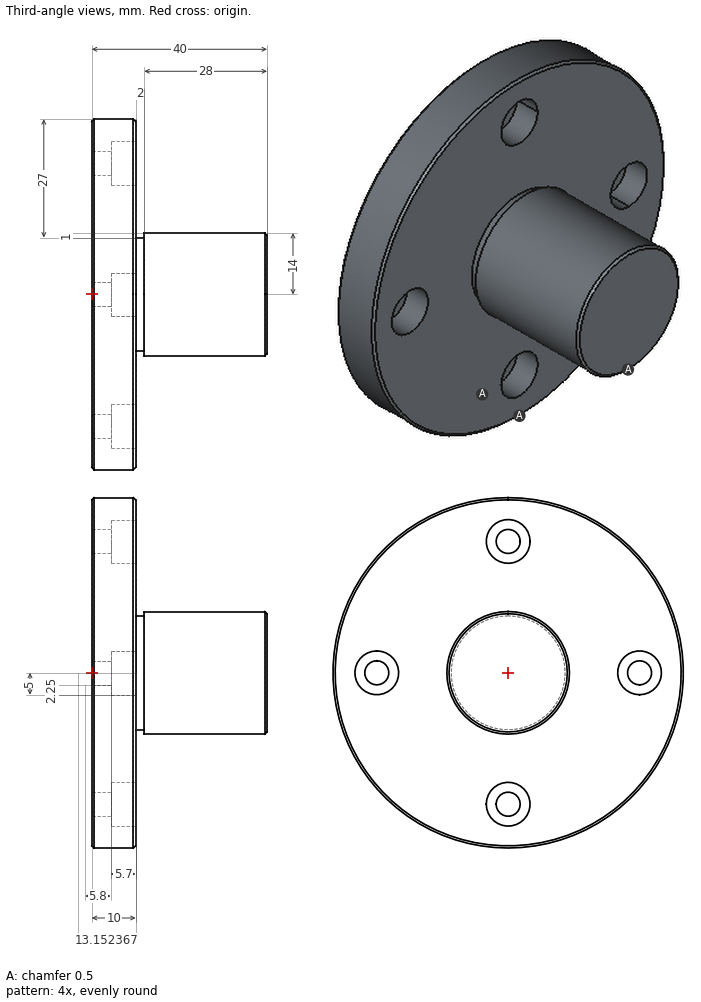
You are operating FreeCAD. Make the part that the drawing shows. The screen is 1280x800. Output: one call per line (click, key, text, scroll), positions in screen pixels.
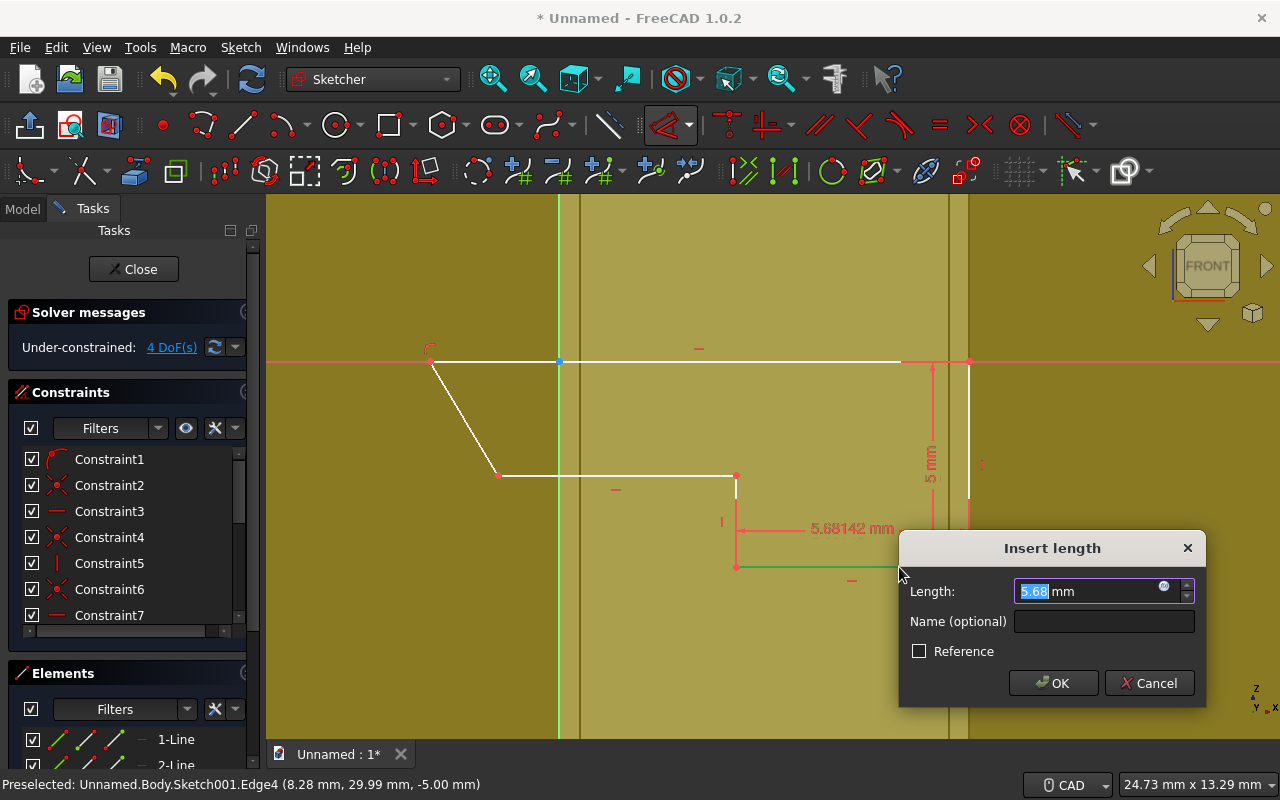
text(5.7)
key(Return)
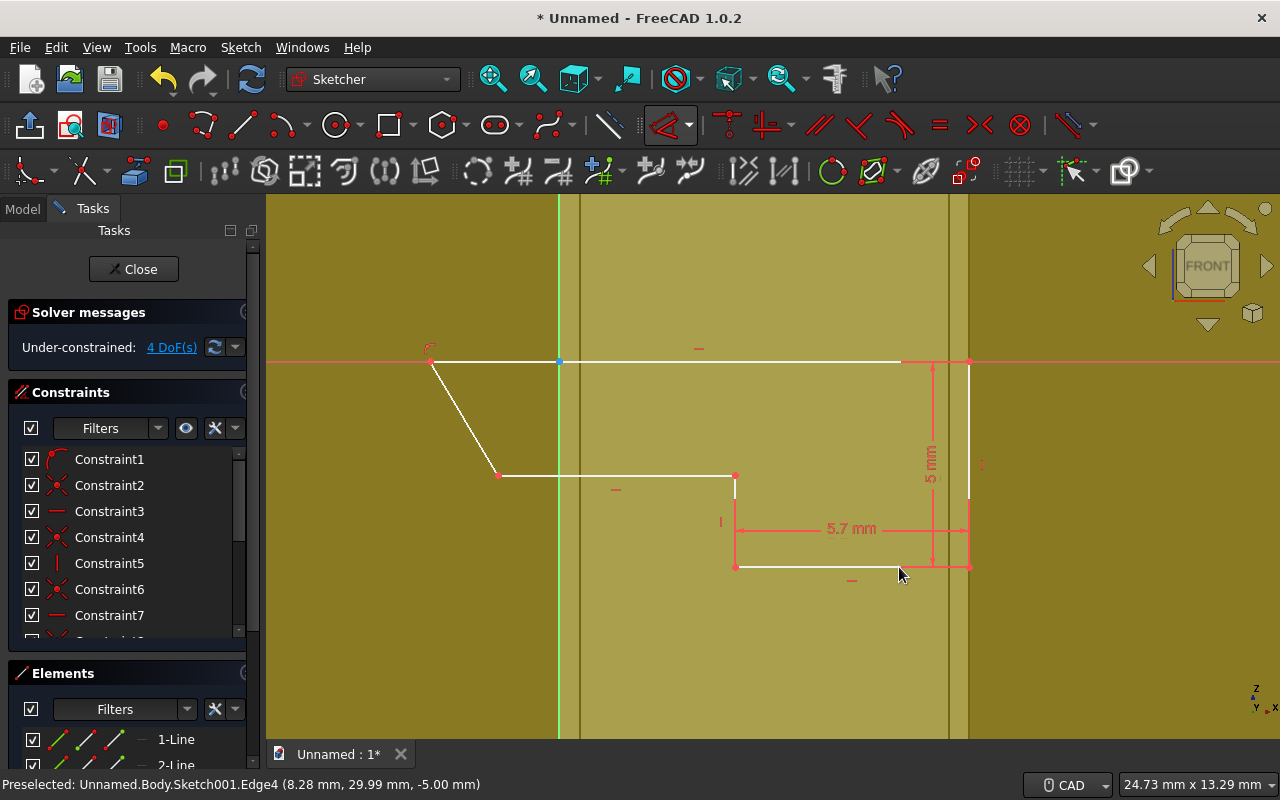
click(664, 476)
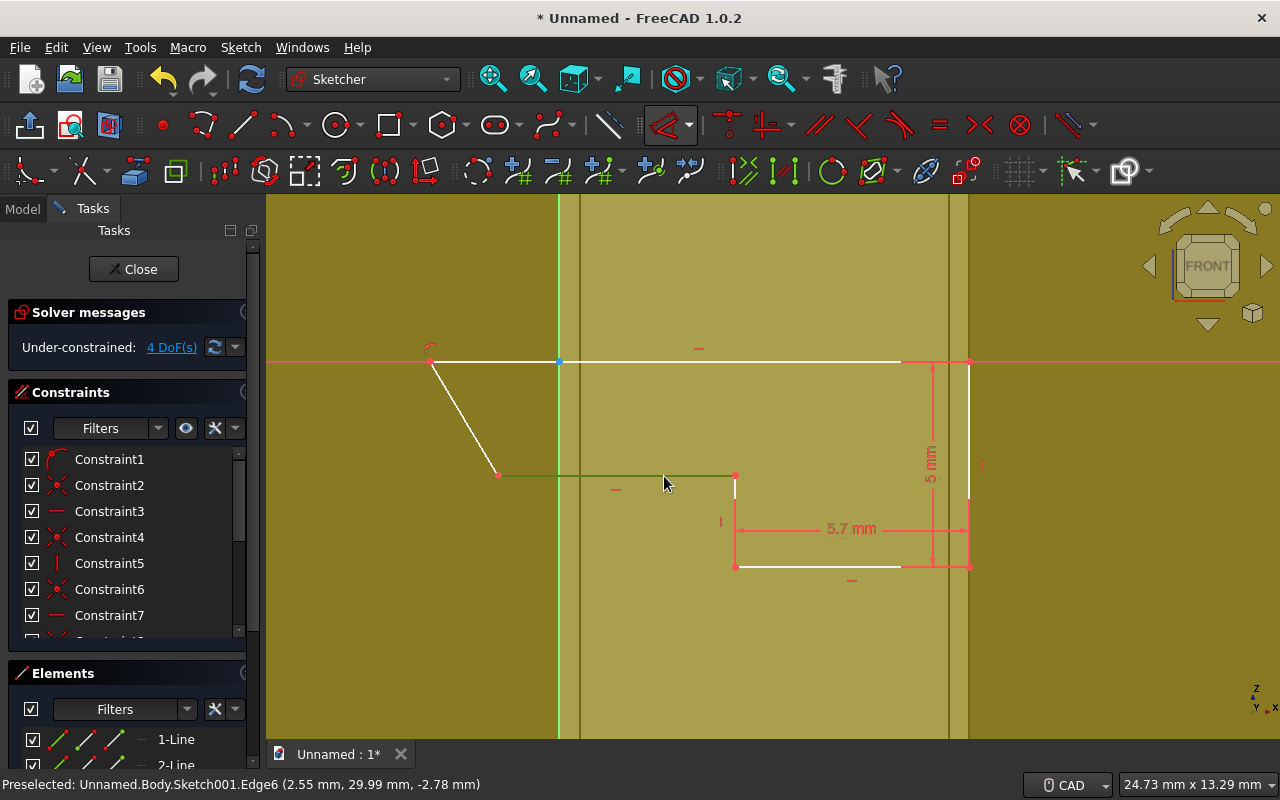
click(692, 126)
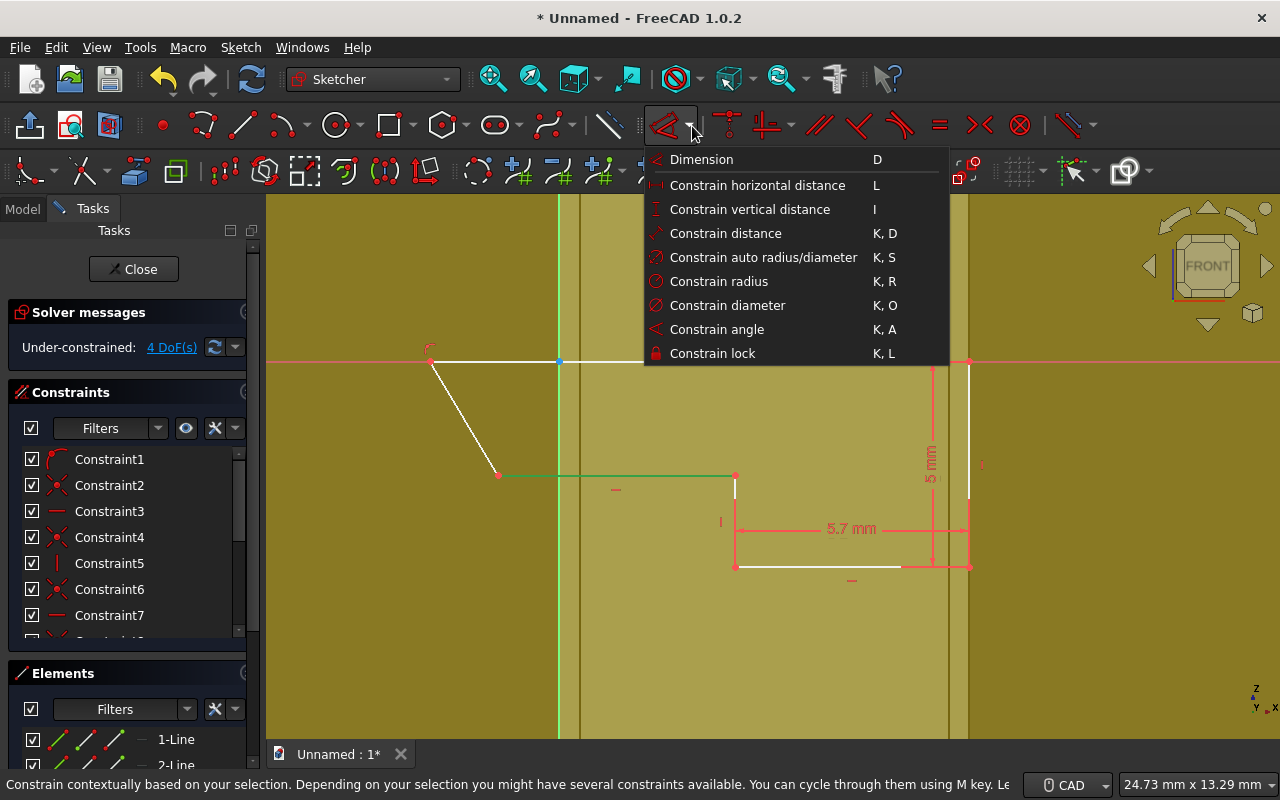
click(797, 185)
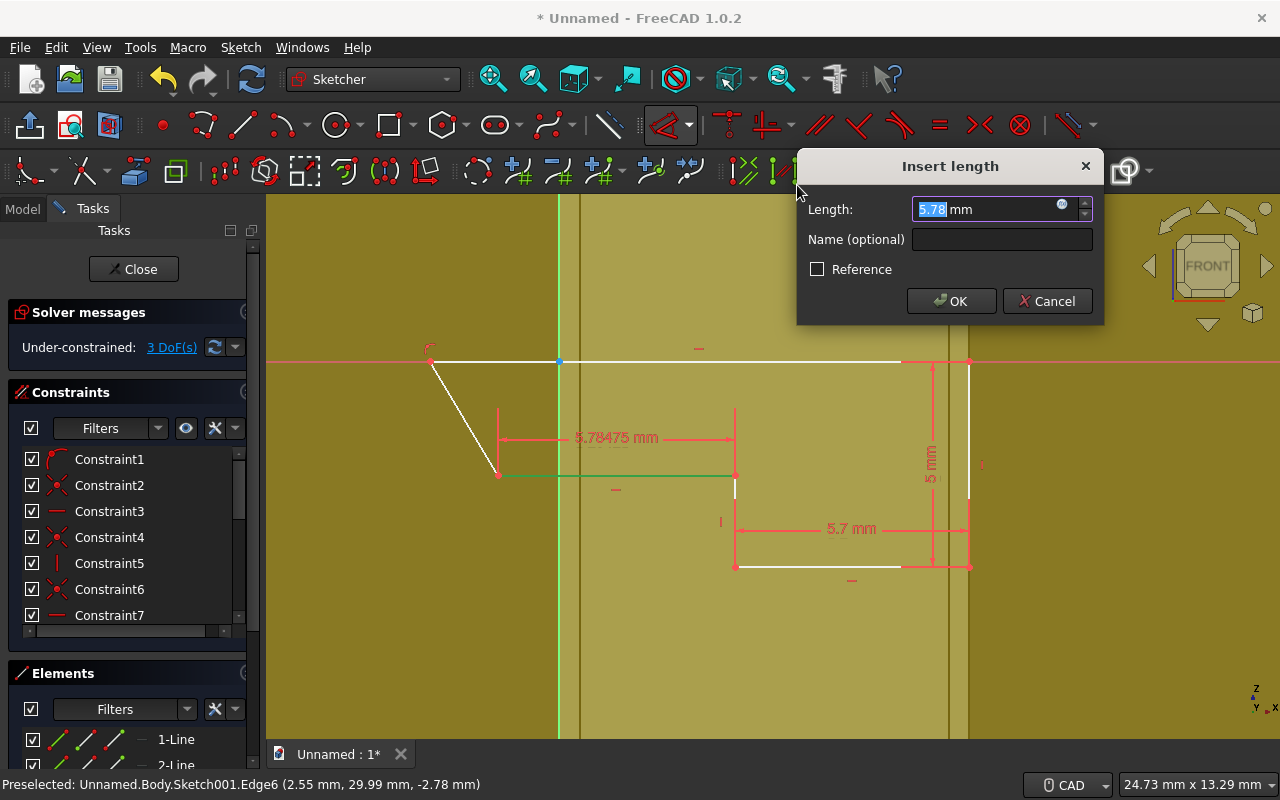
text(5.8)
key(Return)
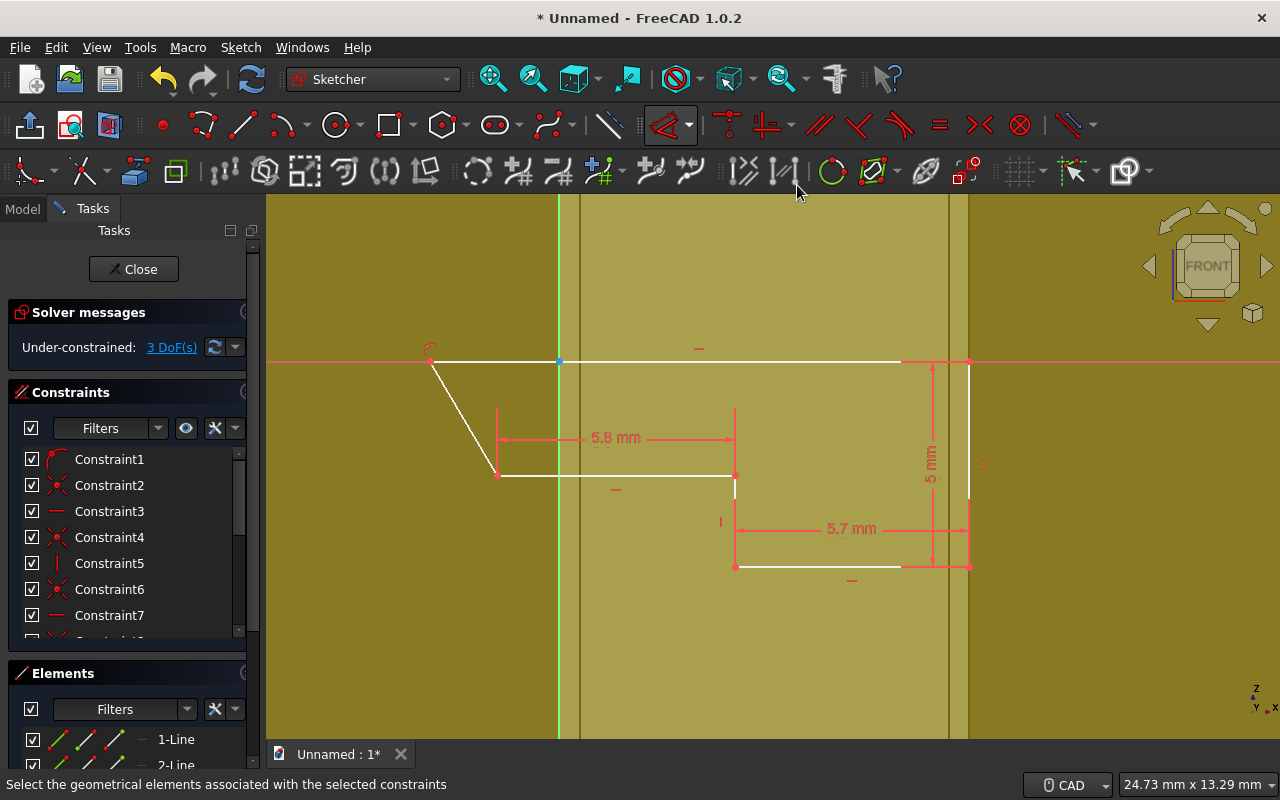
click(969, 362)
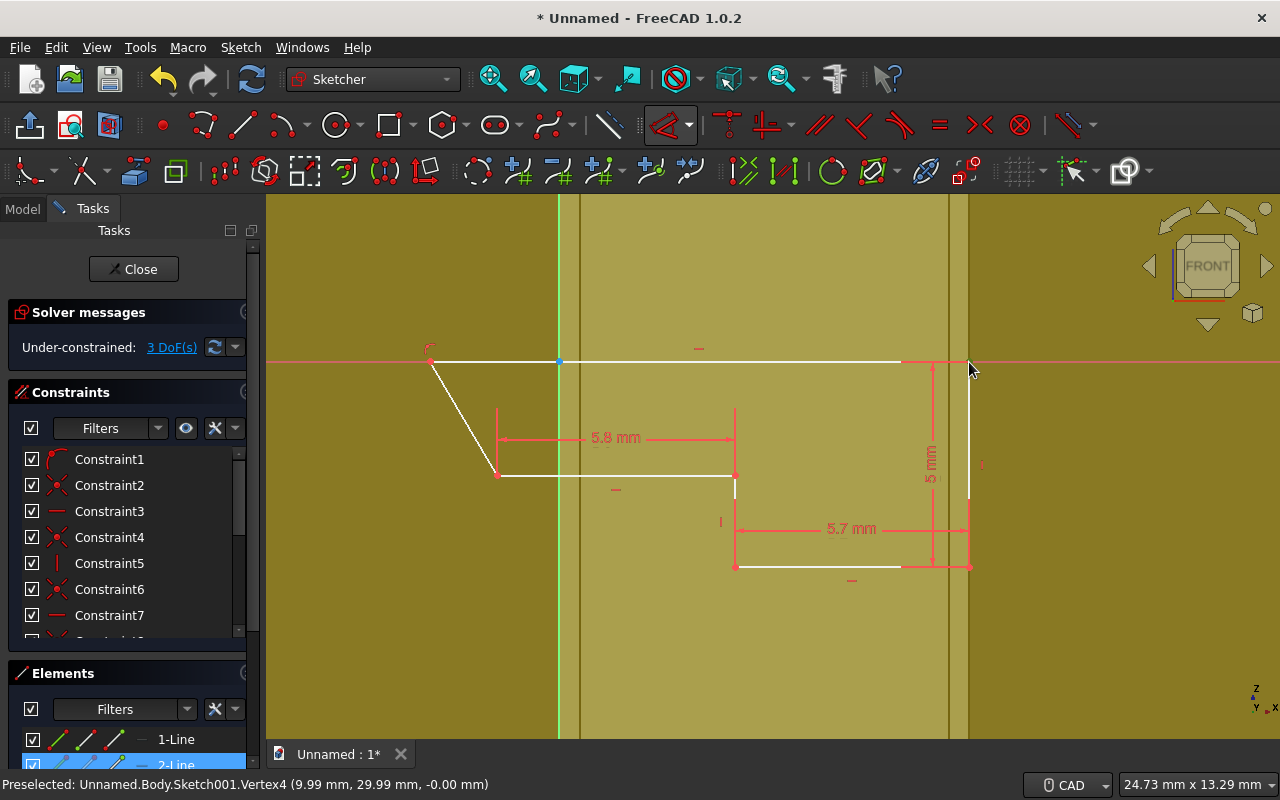
key(l)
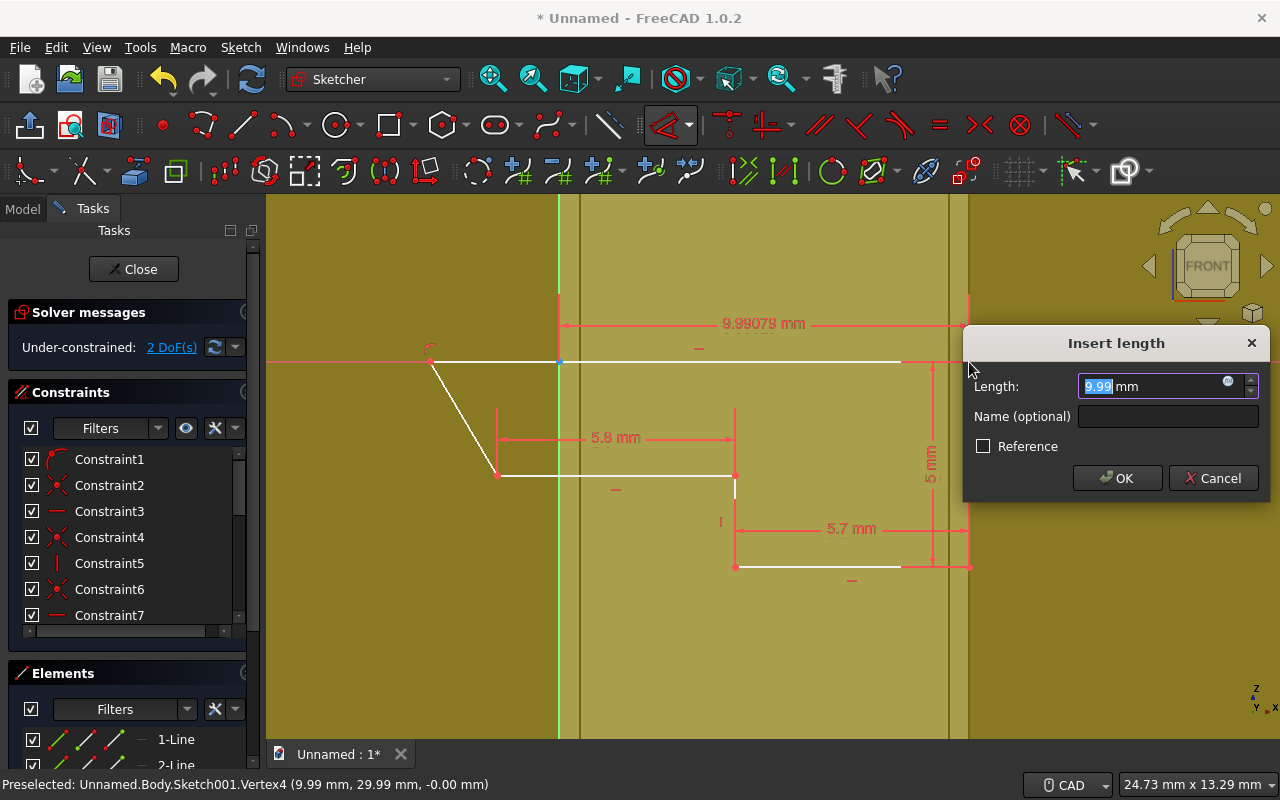
text(10)
key(Return)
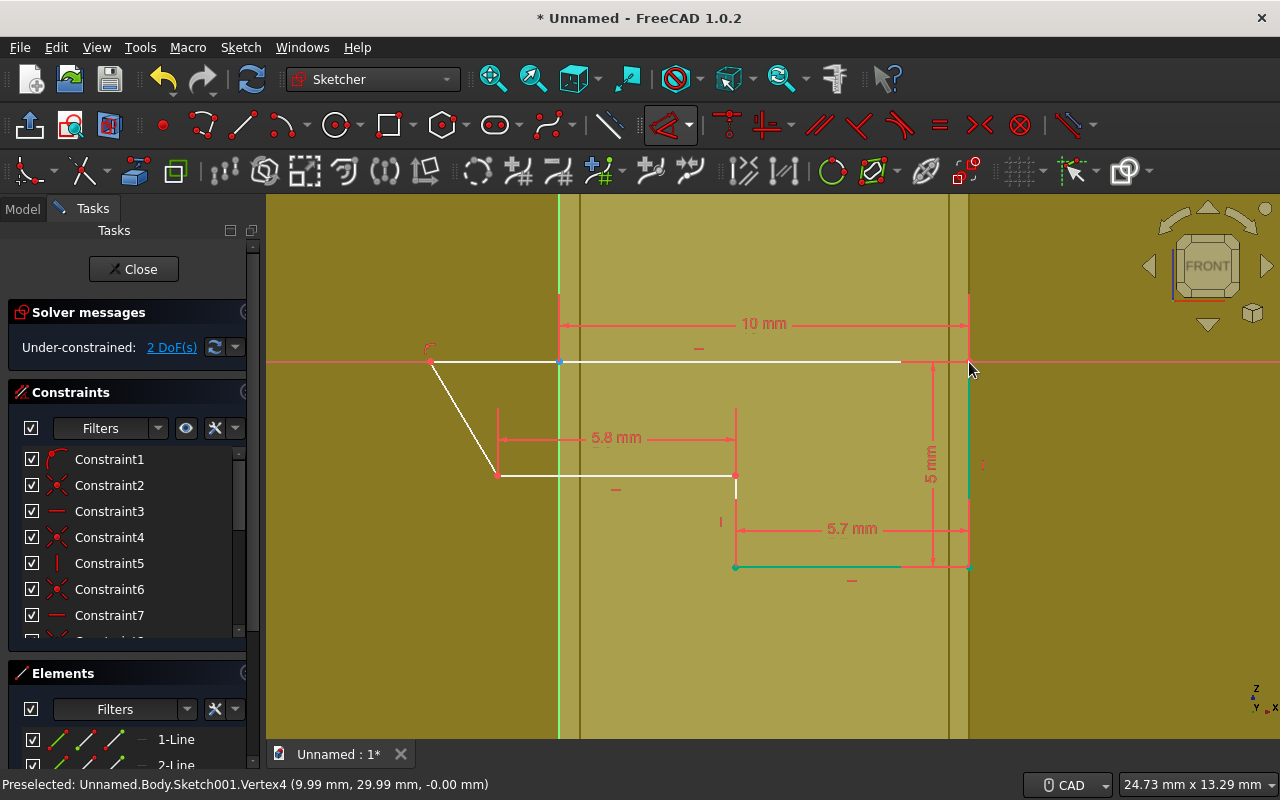
click(736, 540)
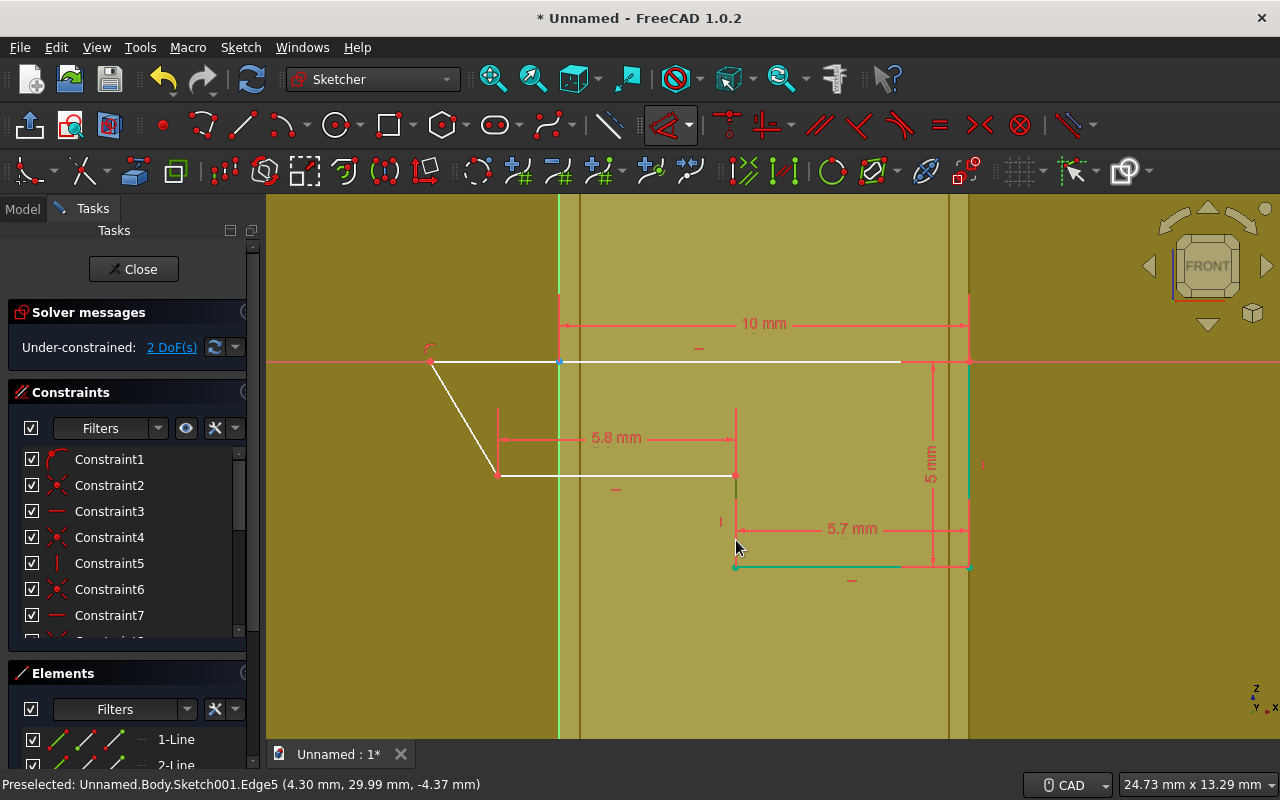
key(i)